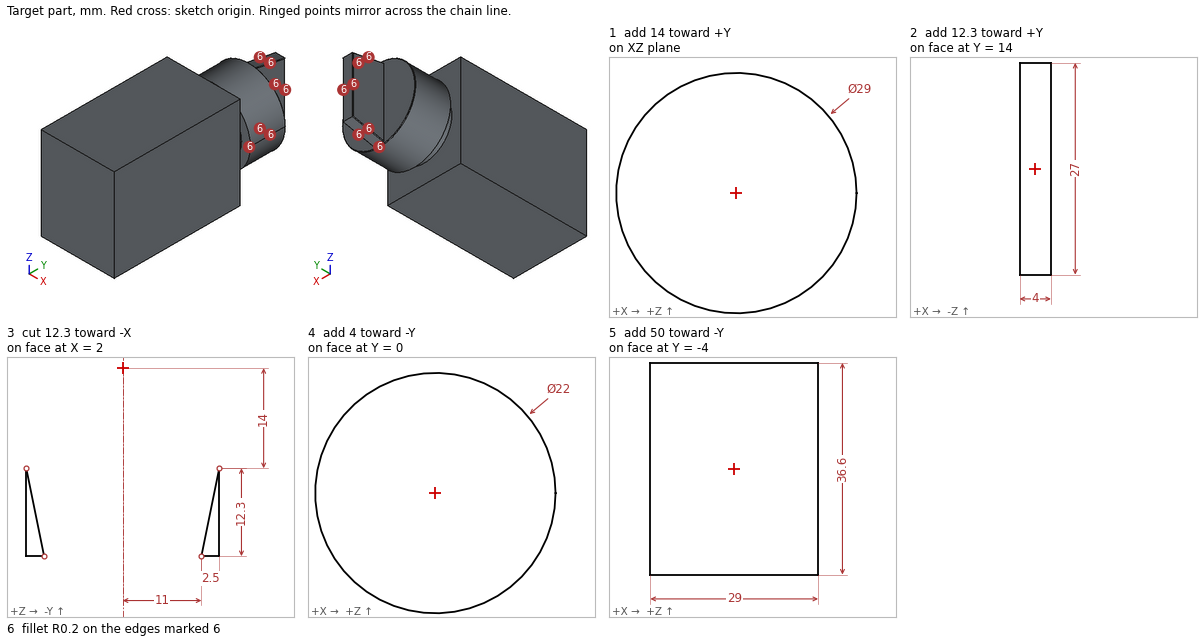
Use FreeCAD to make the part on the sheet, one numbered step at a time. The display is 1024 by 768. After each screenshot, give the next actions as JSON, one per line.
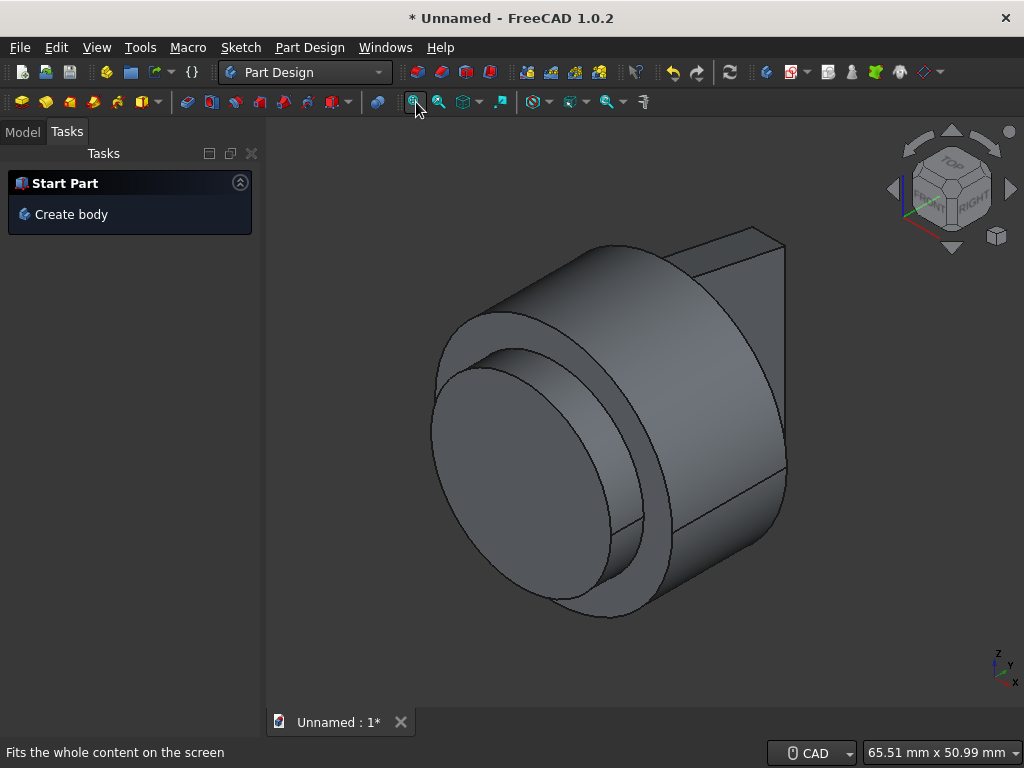
{"action": "left_click", "coordinate": [521, 483]}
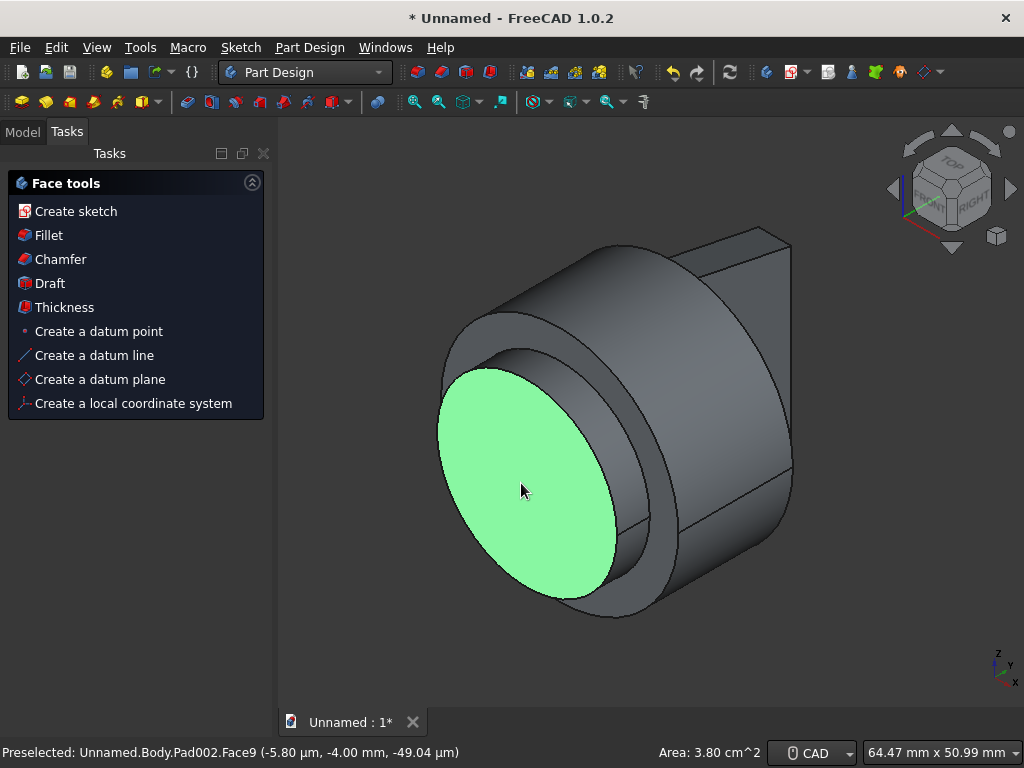
{"action": "left_click", "coordinate": [792, 72]}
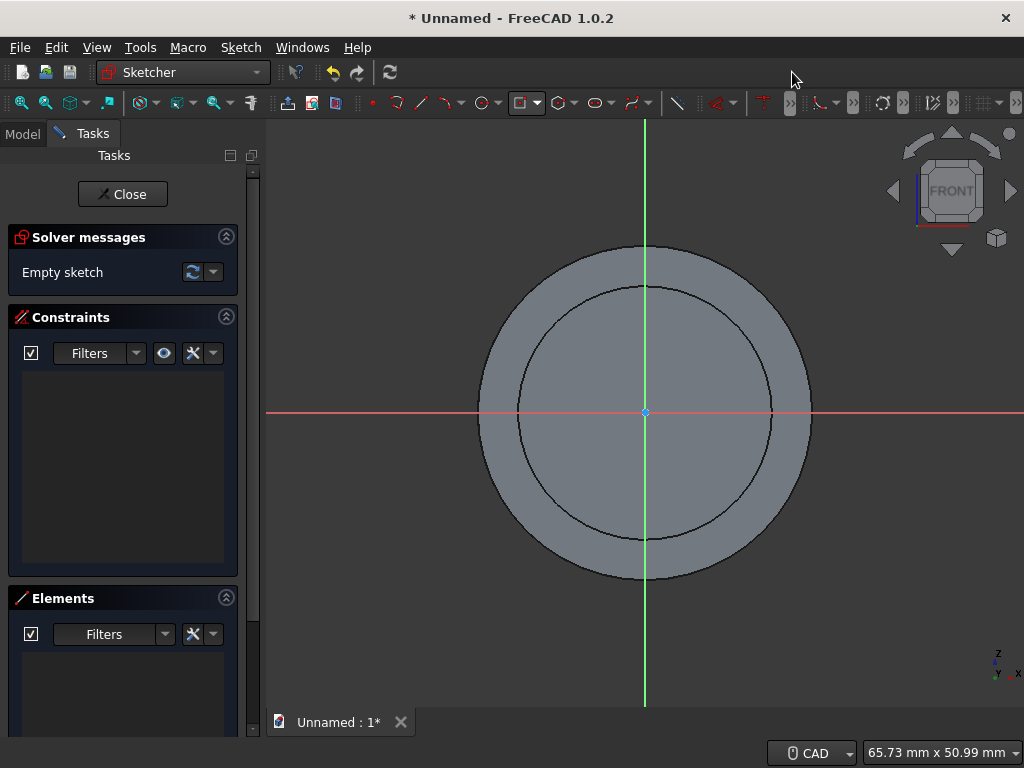
{"action": "left_click", "coordinate": [520, 104]}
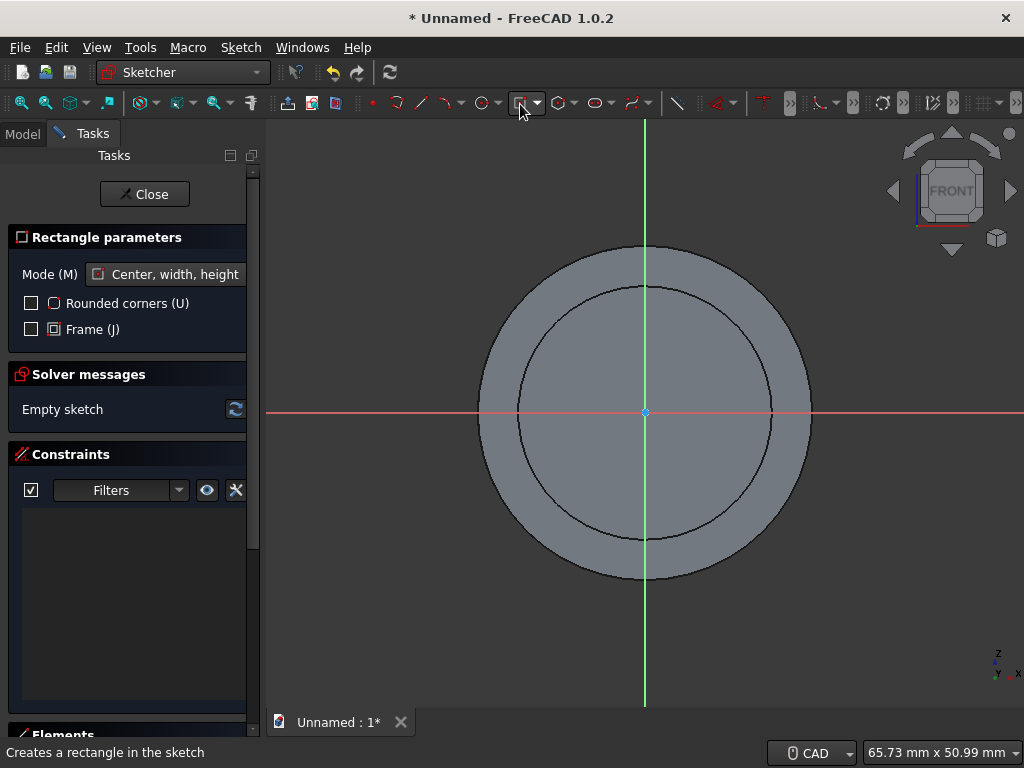
{"action": "left_click", "coordinate": [645, 413]}
{"action": "mouse_move", "coordinate": [812, 202]}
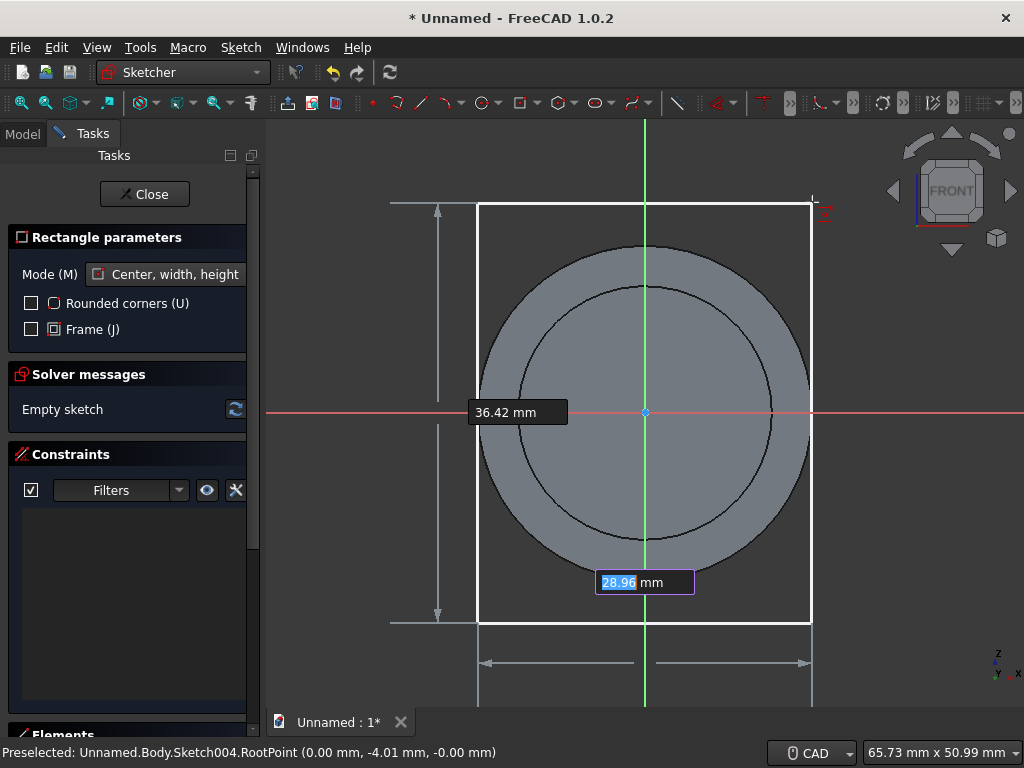
{"action": "type", "text": "29"}
{"action": "key", "text": "Tab"}
{"action": "type", "text": "36.6"}
{"action": "key", "text": "Return"}
{"action": "key", "text": "Escape"}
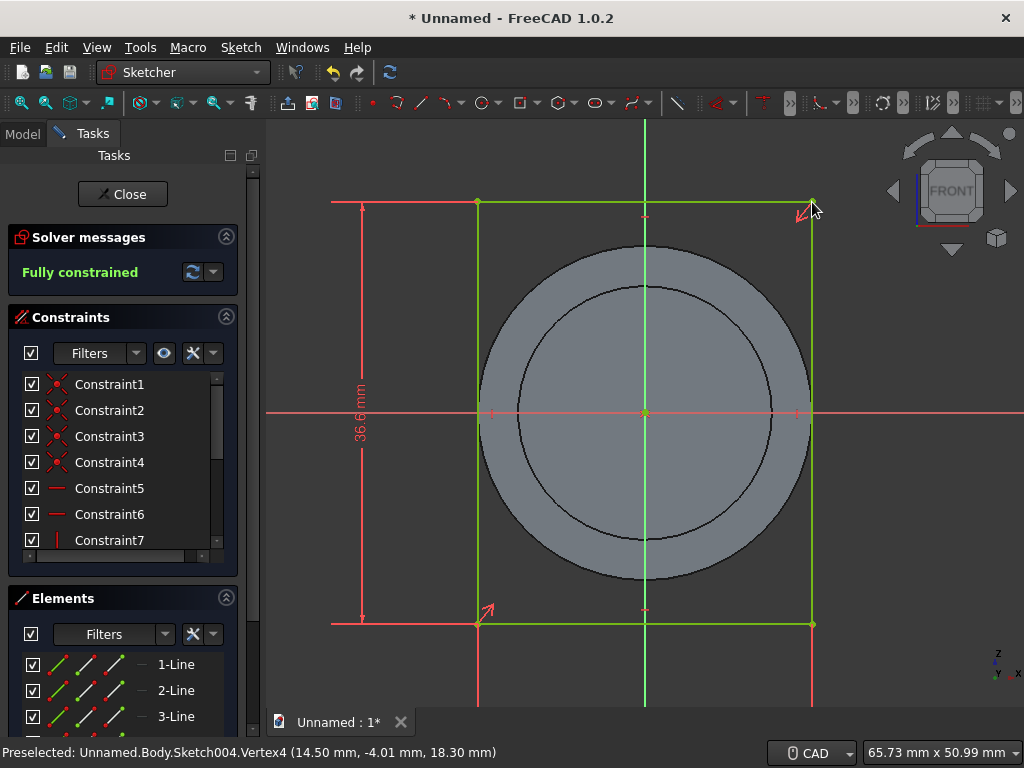
{"action": "left_click", "coordinate": [123, 194]}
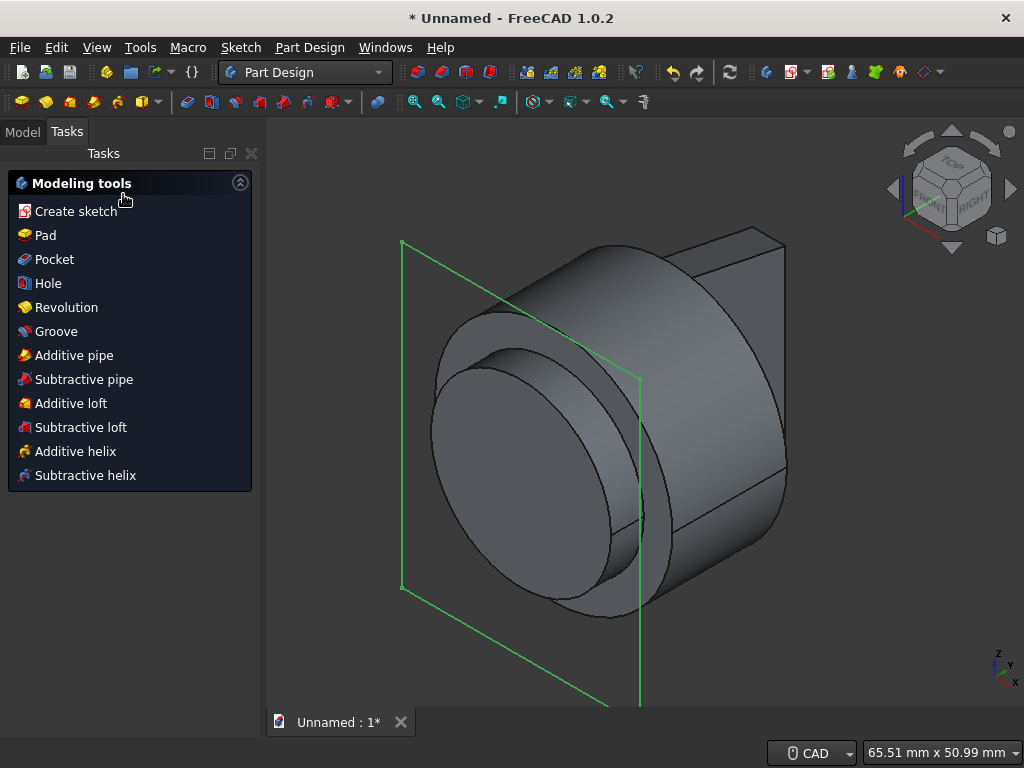
{"action": "left_click", "coordinate": [22, 102]}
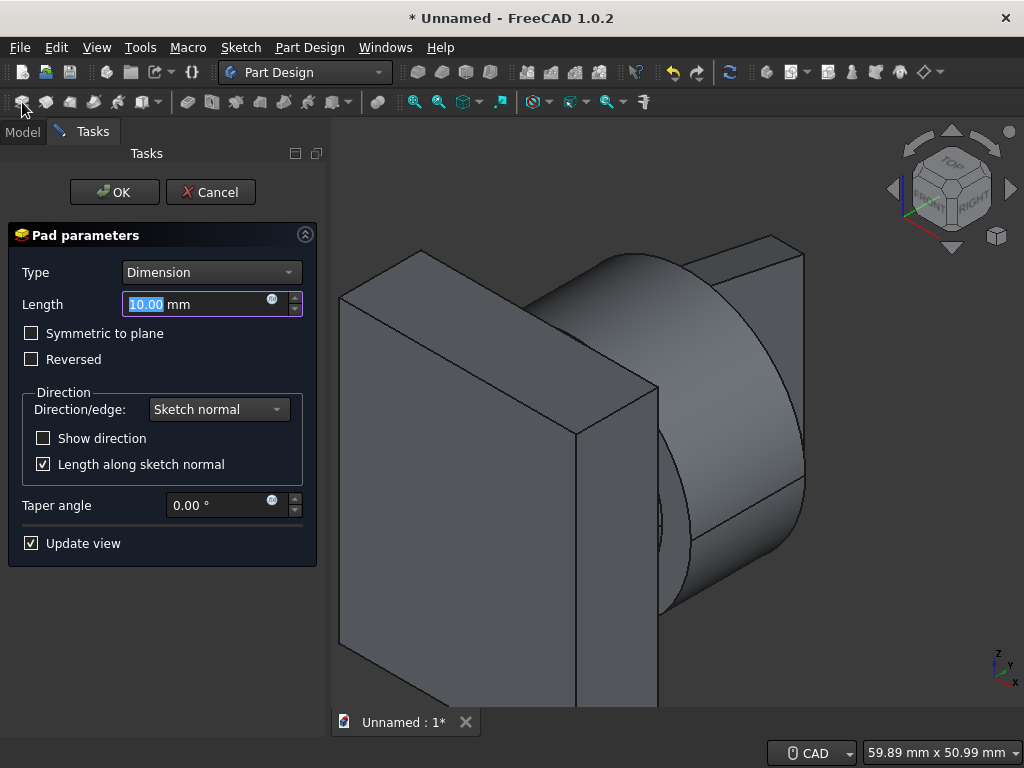
{"action": "type", "text": "50"}
{"action": "key", "text": "Tab"}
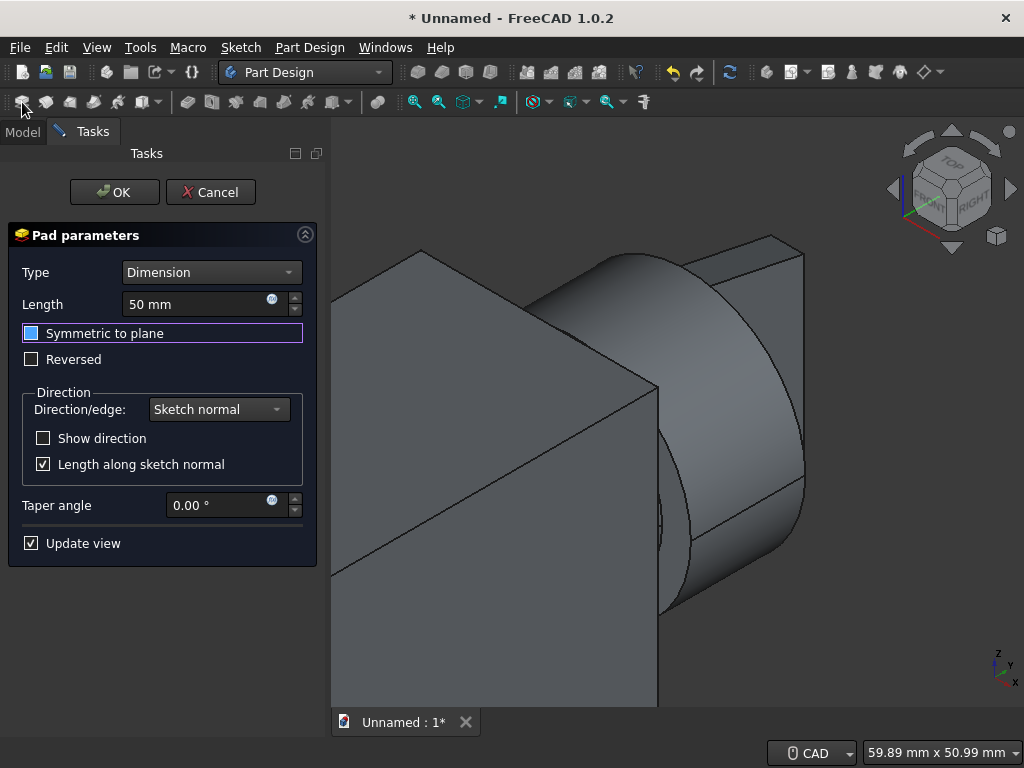
{"action": "left_click", "coordinate": [115, 192]}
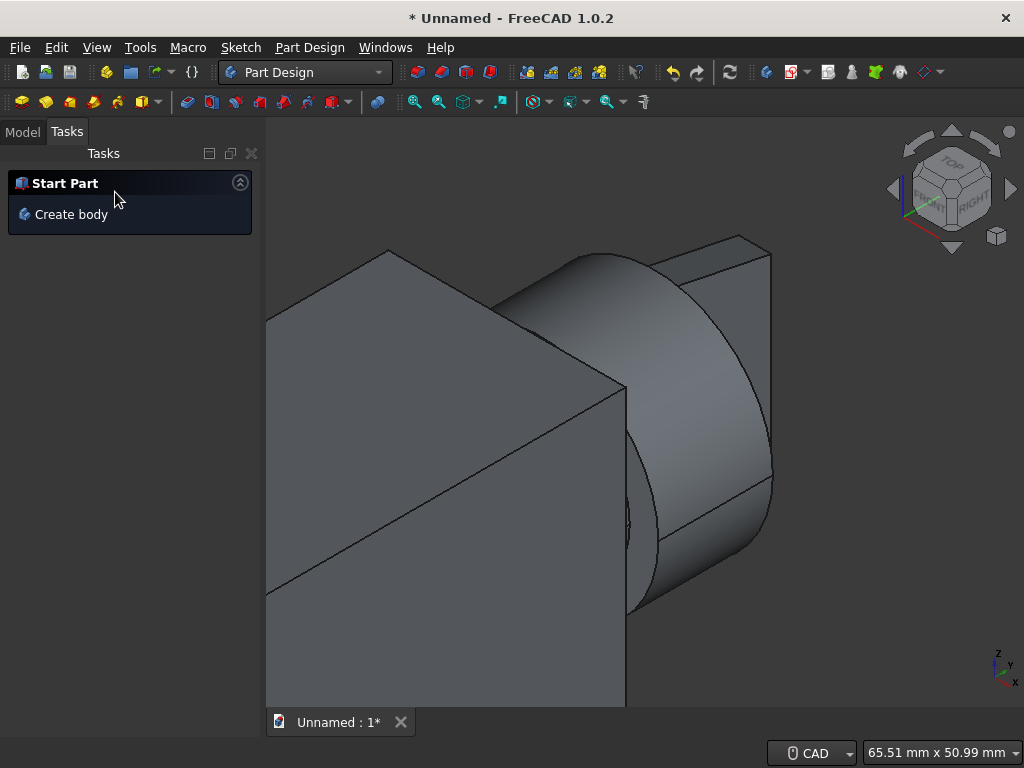
{"action": "left_click", "coordinate": [416, 102]}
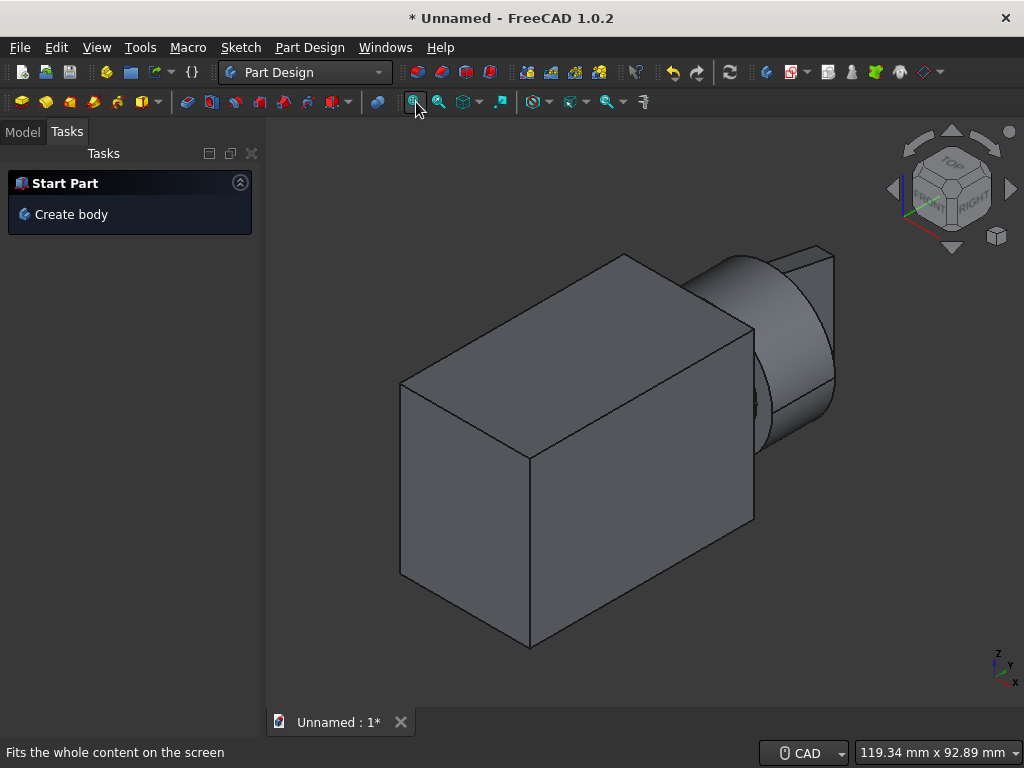
{"action": "left_click", "coordinate": [807, 264]}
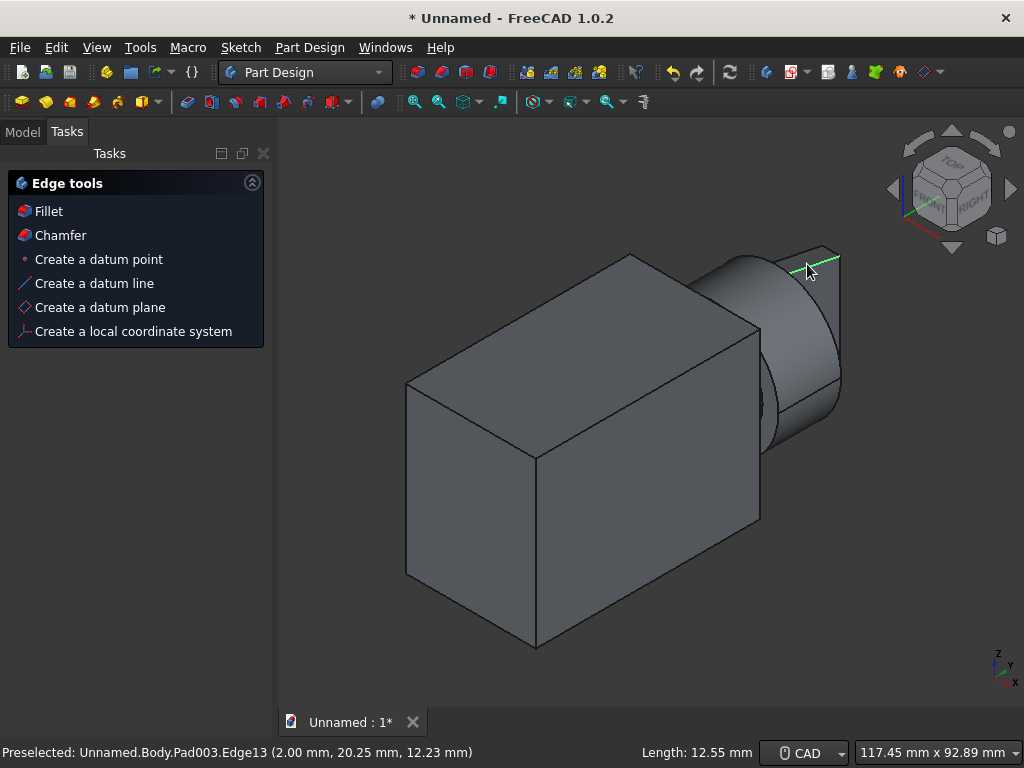
{"action": "key", "text": "2"}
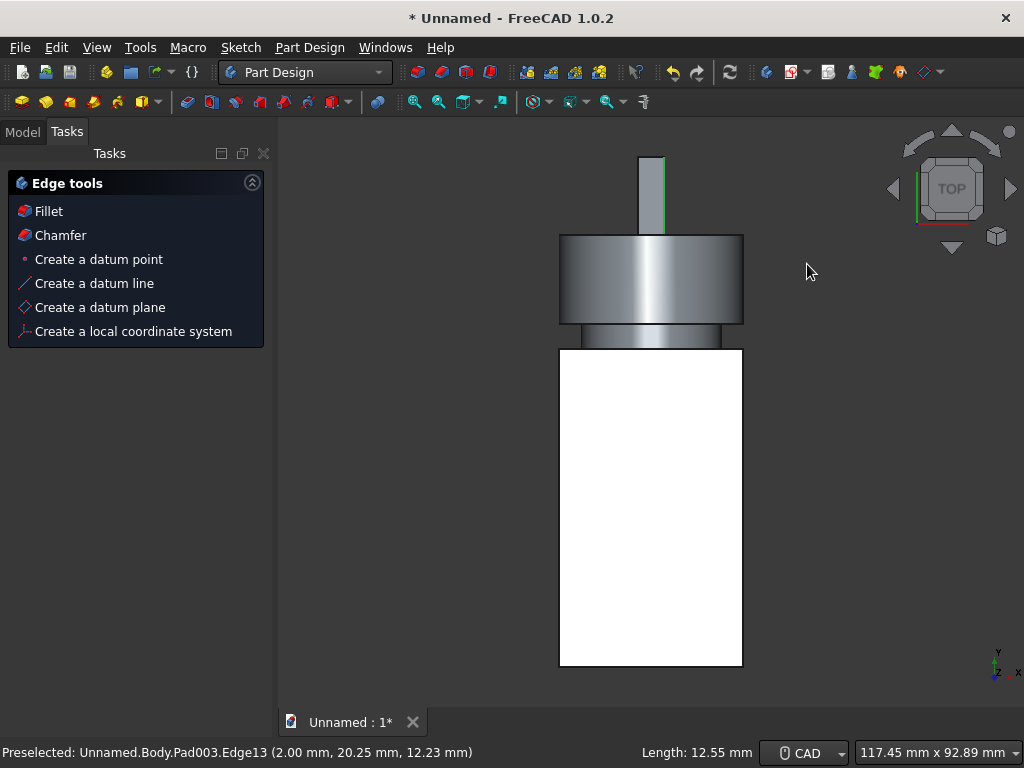
{"action": "left_click", "coordinate": [638, 195], "text": "ctrl"}